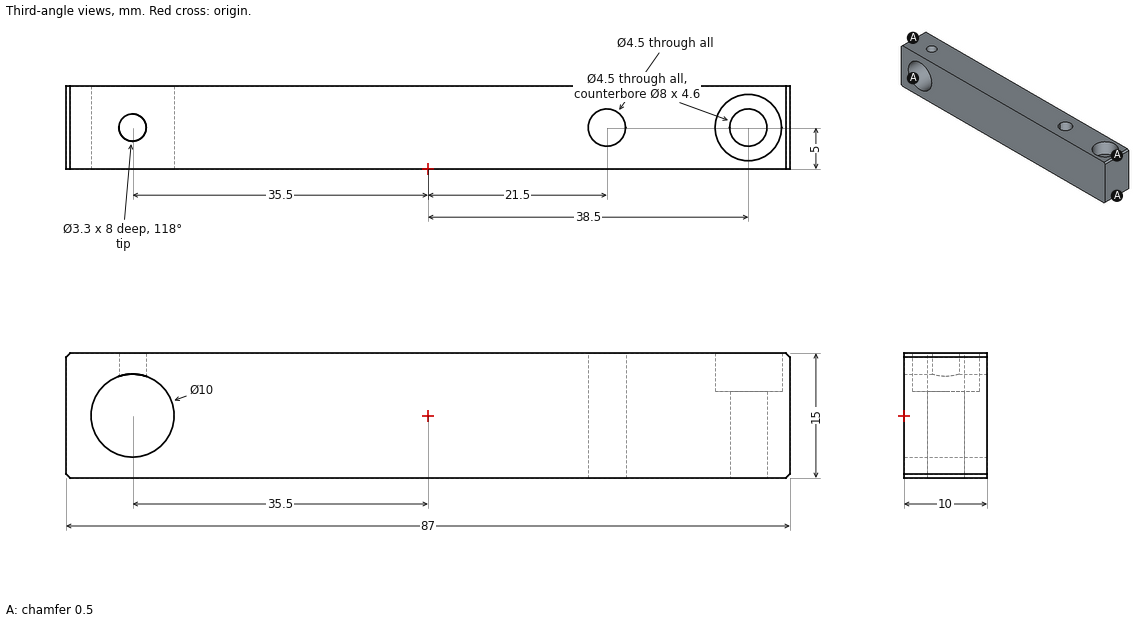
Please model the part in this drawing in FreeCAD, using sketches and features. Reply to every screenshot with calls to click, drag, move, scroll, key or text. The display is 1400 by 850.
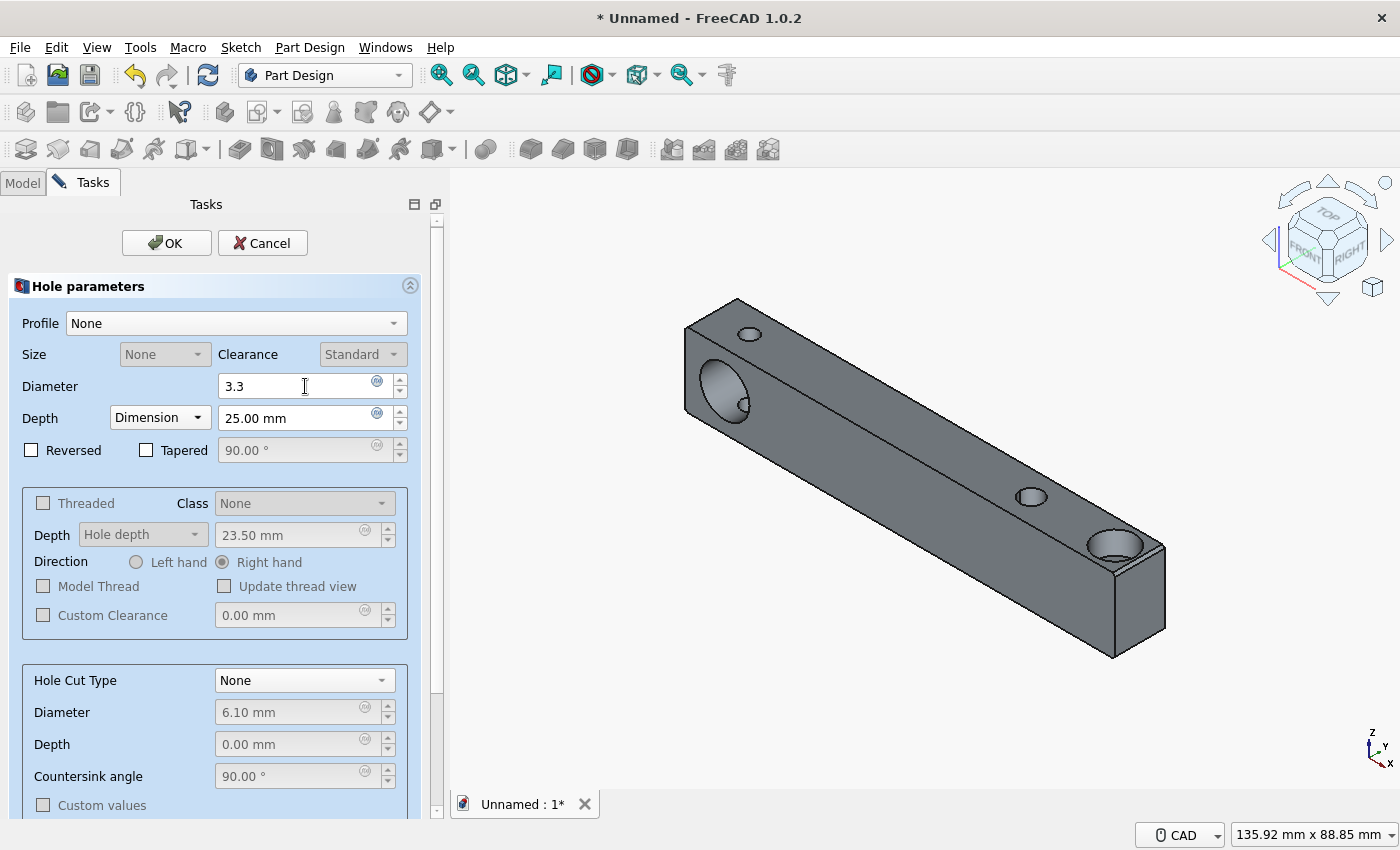
triple_click(305, 418)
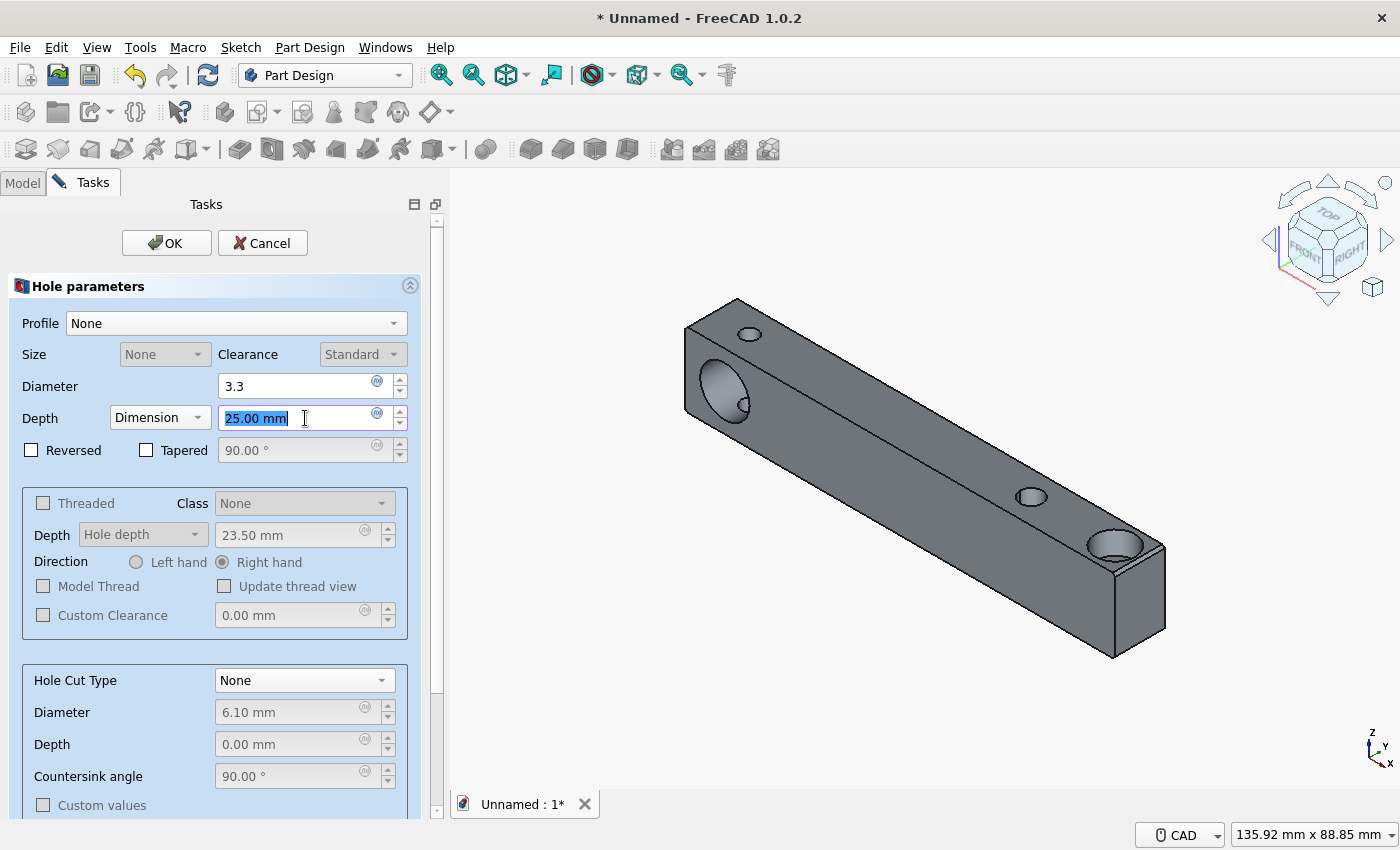
text(8)
key(Tab)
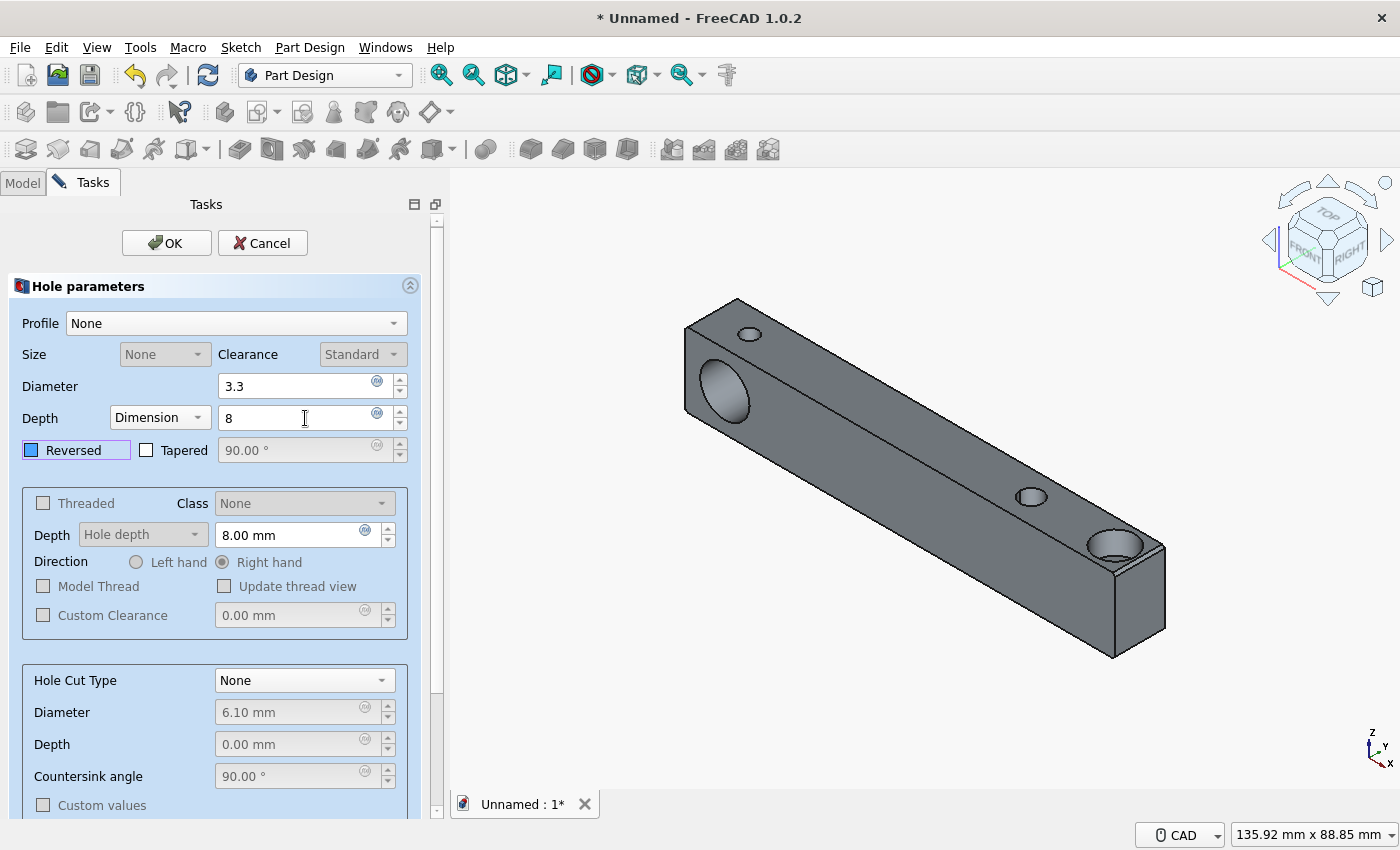
click(167, 243)